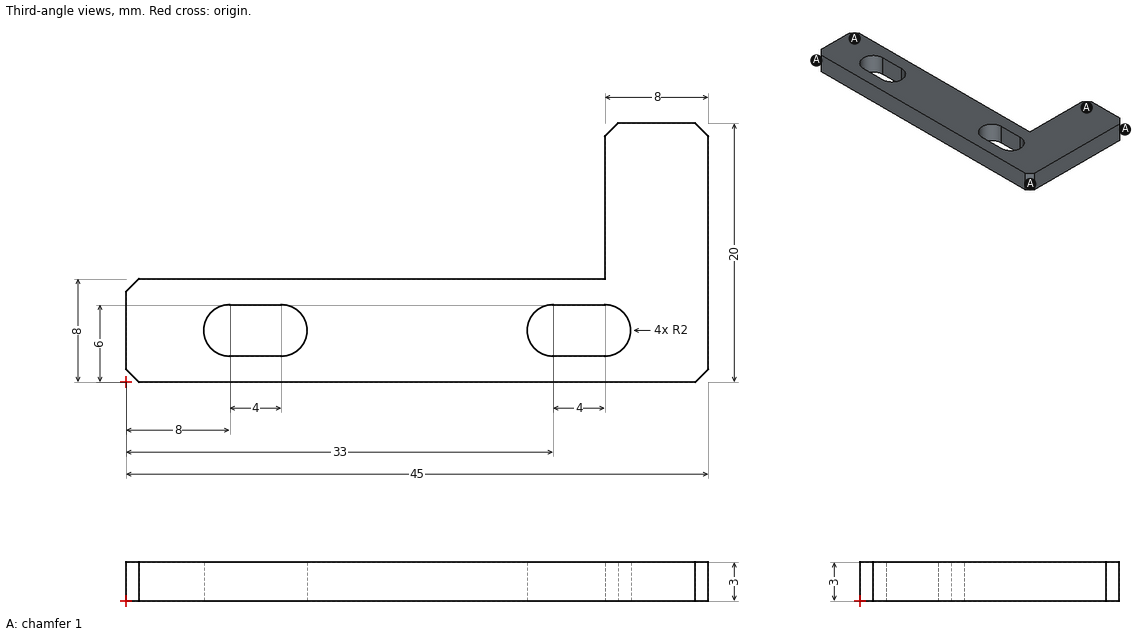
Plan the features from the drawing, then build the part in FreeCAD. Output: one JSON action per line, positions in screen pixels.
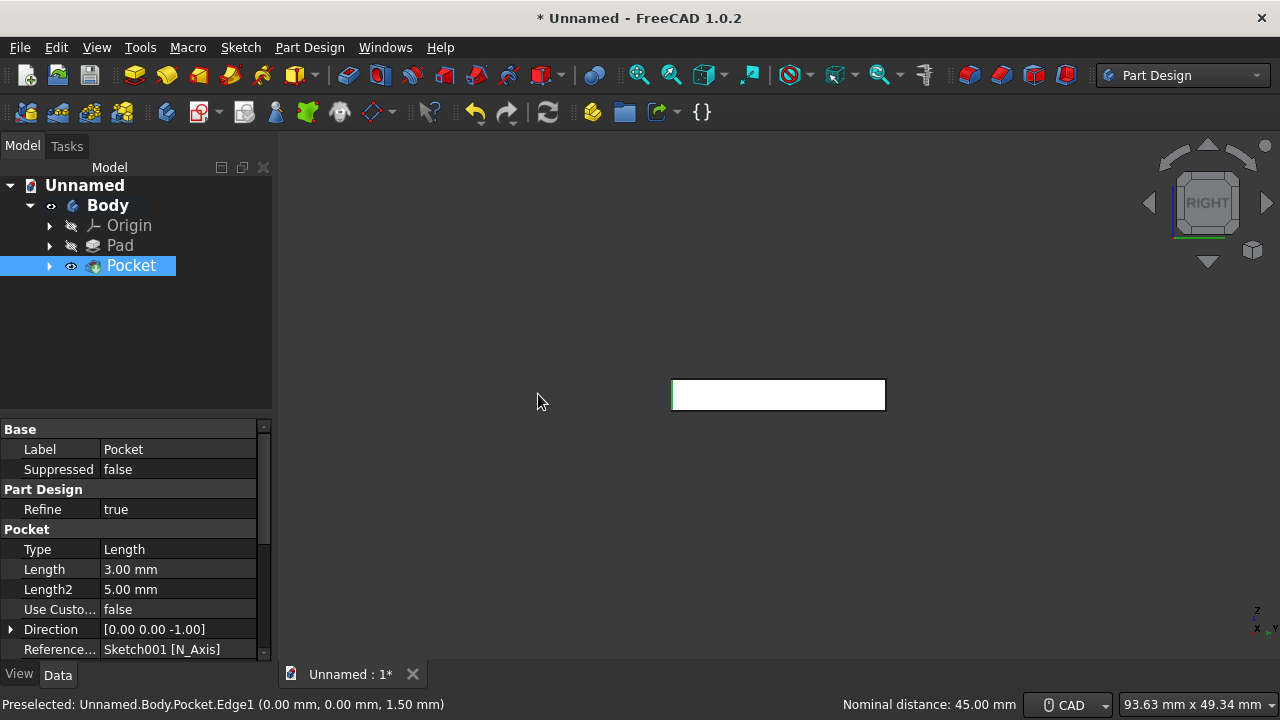
{"action": "left_click", "coordinate": [640, 76]}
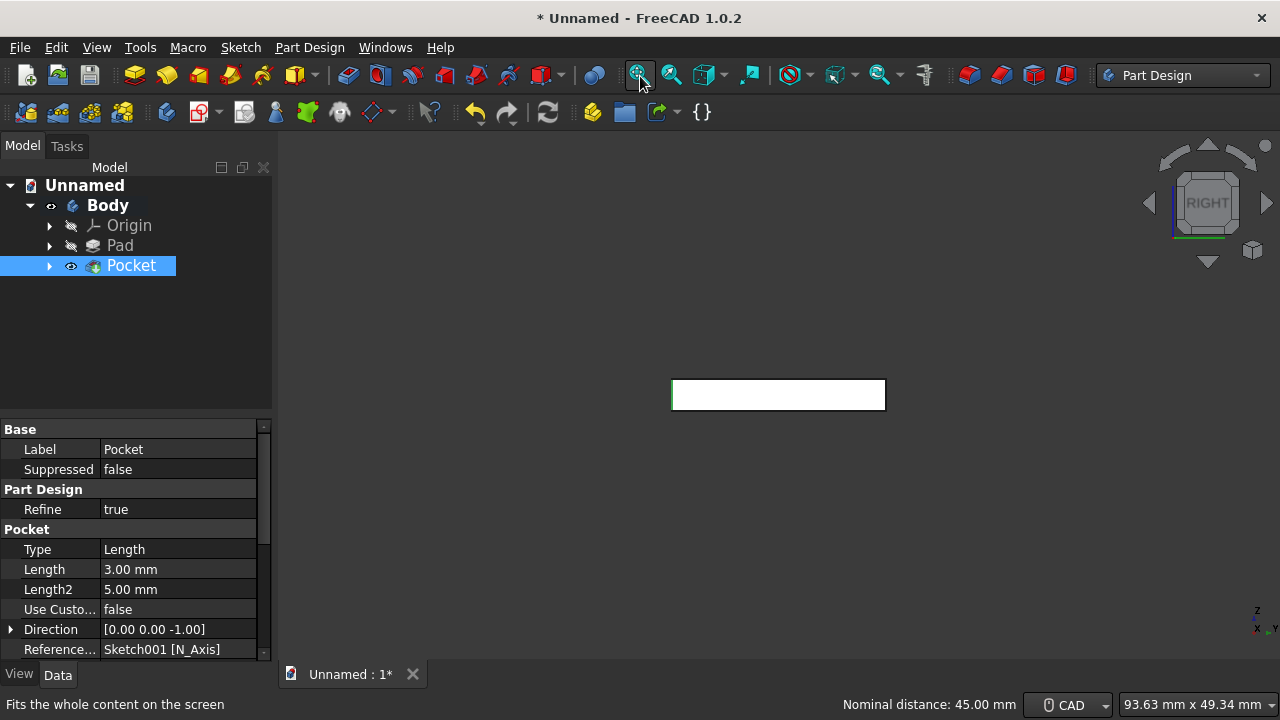
{"action": "left_click", "coordinate": [886, 394], "text": "ctrl"}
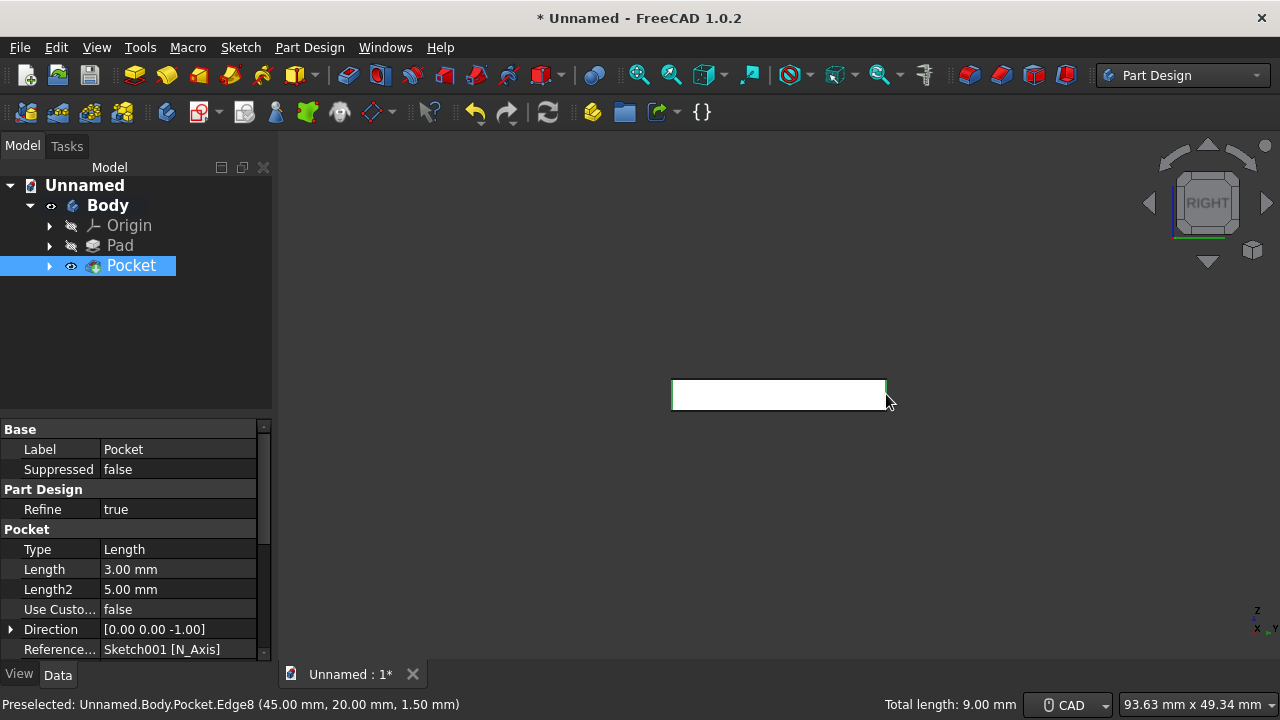
{"action": "key", "text": "5"}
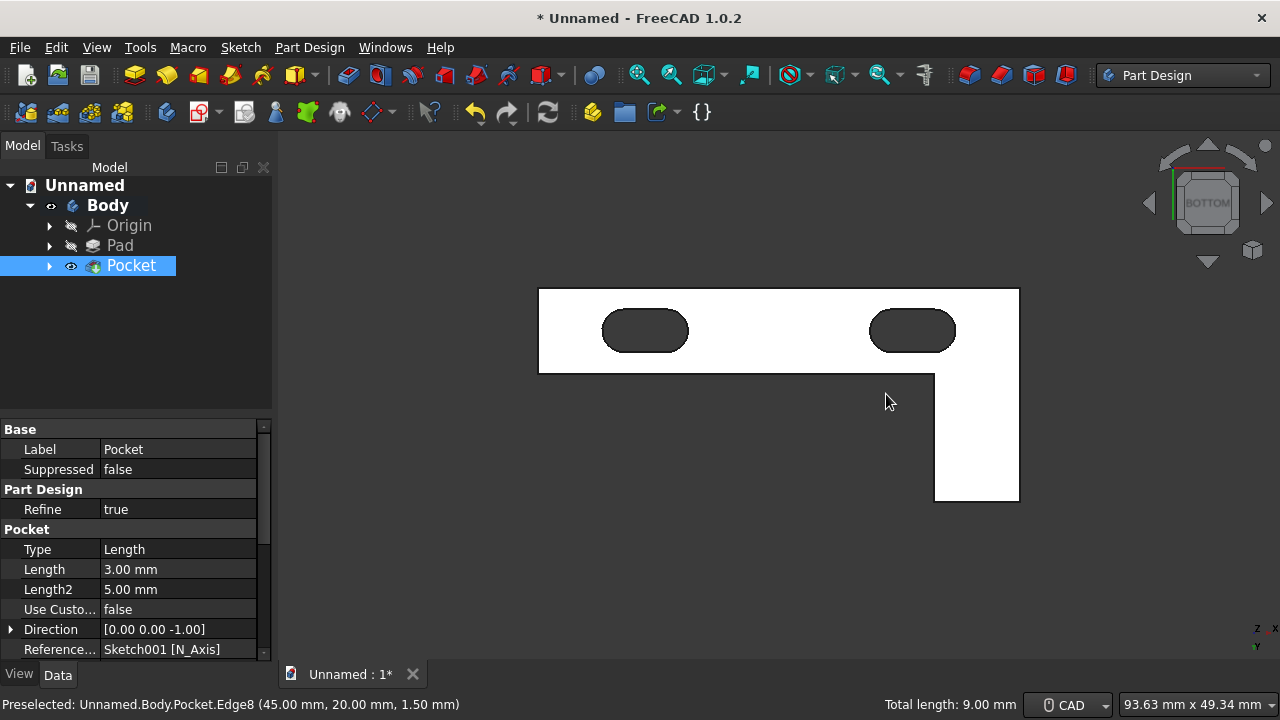
{"action": "key", "text": "4"}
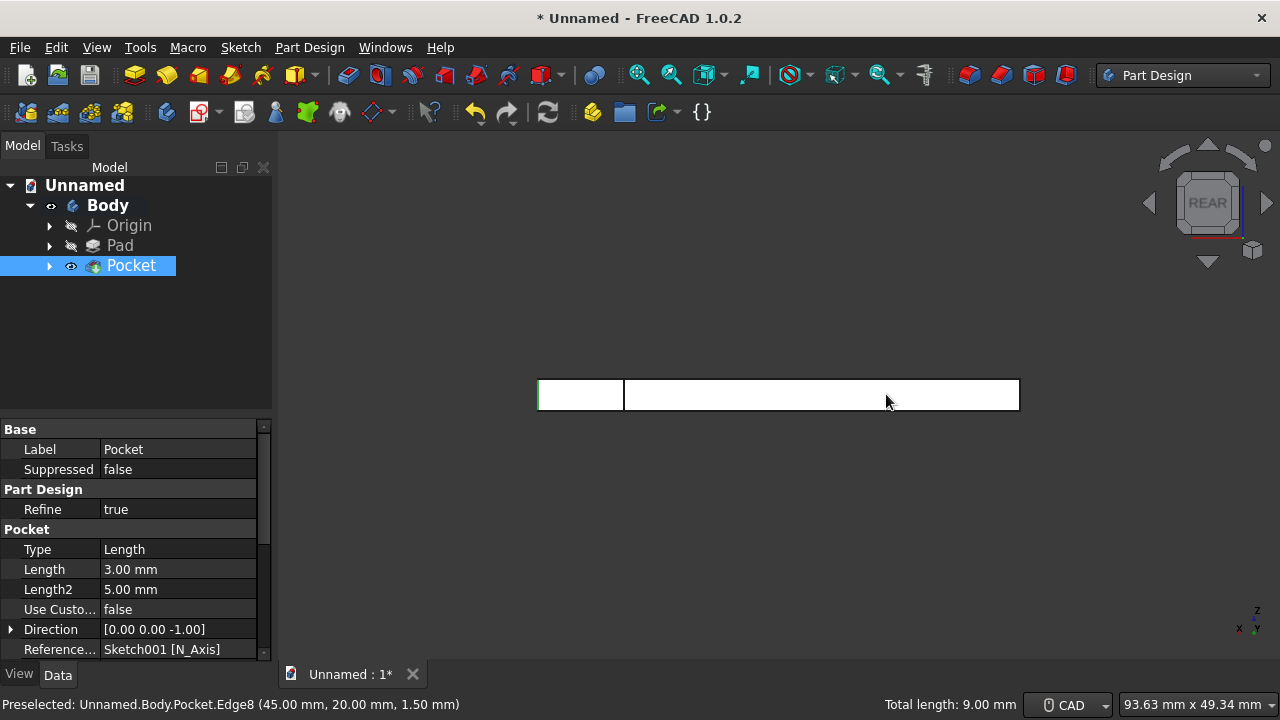
{"action": "left_click", "coordinate": [1020, 394], "text": "ctrl"}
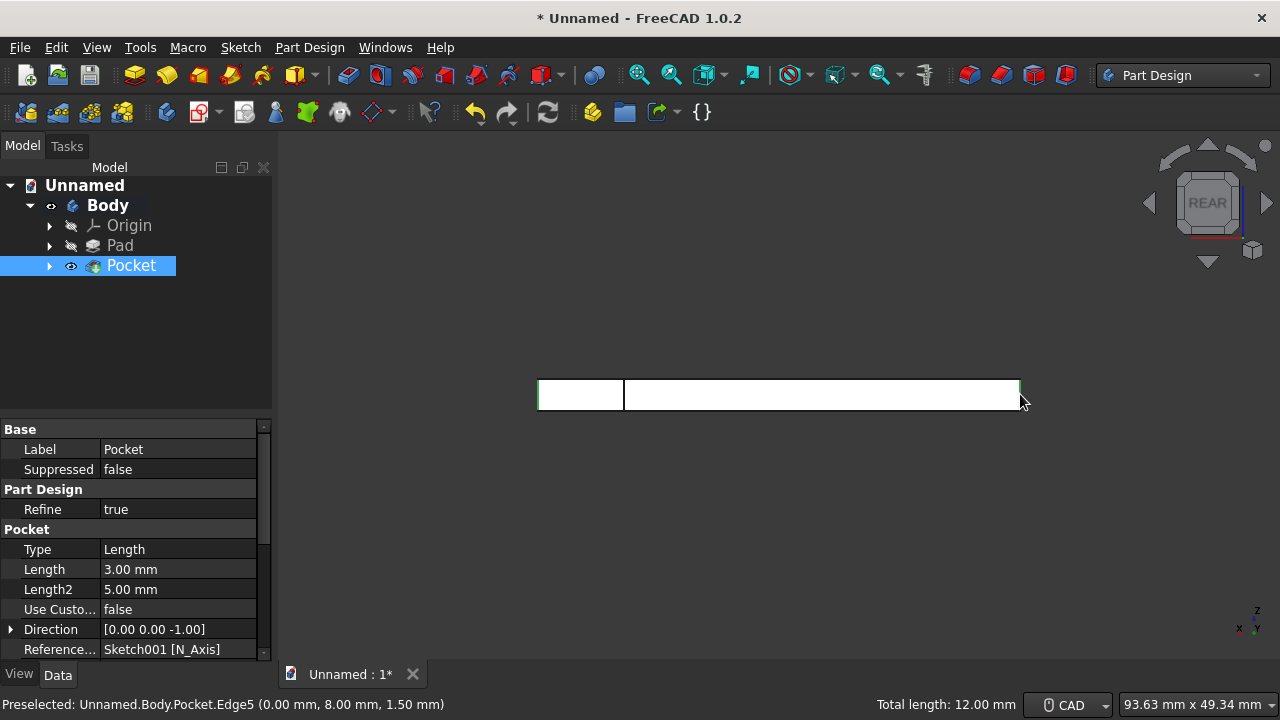
{"action": "left_click", "coordinate": [624, 394], "text": "ctrl"}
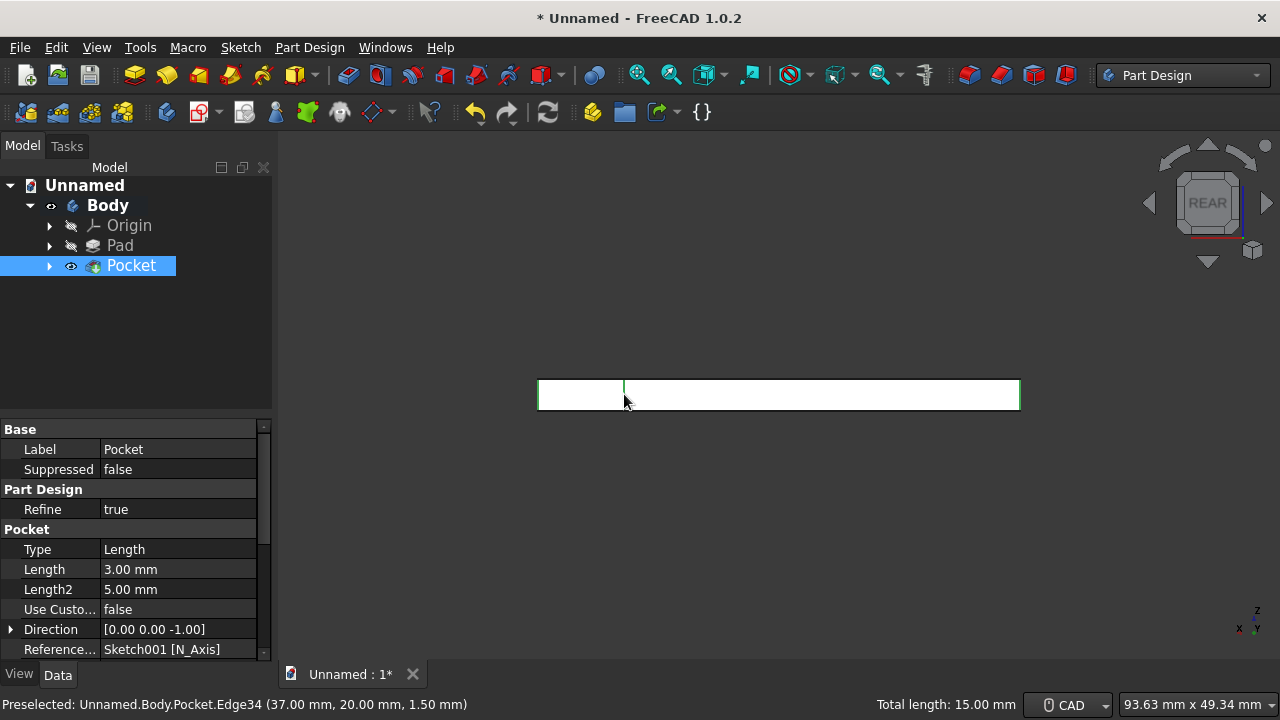
{"action": "left_click", "coordinate": [1002, 76]}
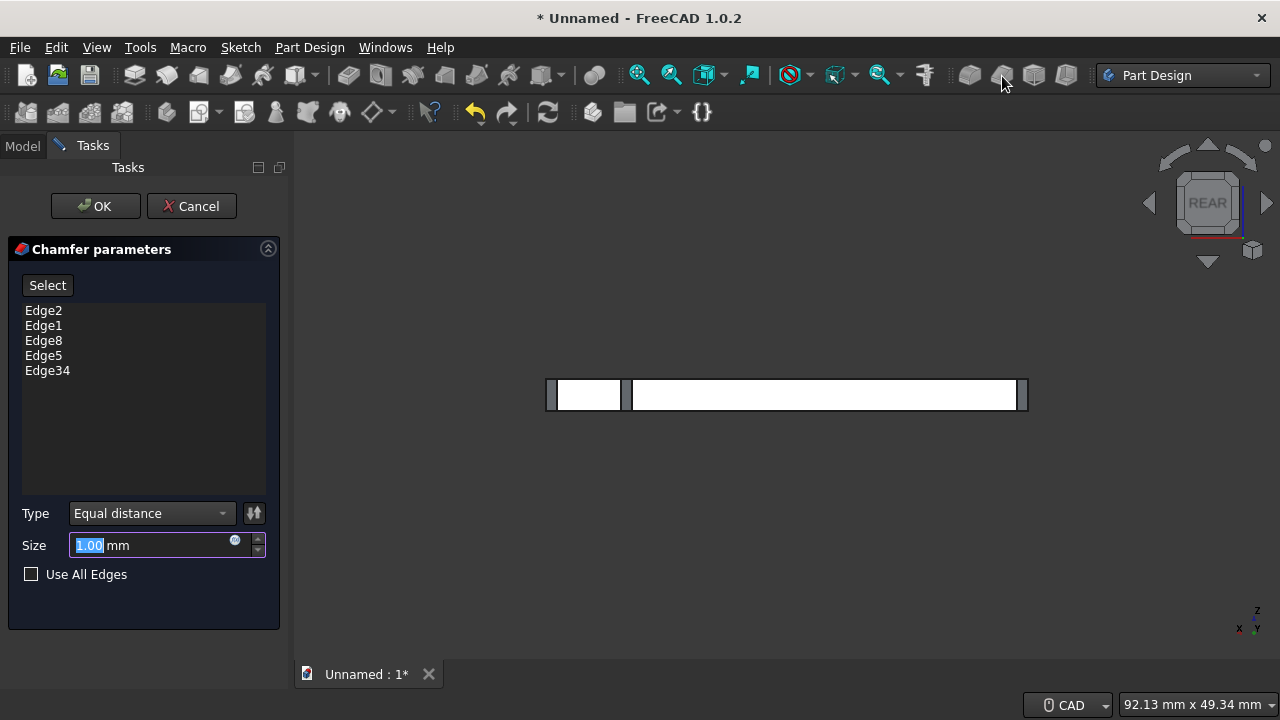
{"action": "type", "text": "1"}
{"action": "key", "text": "Tab"}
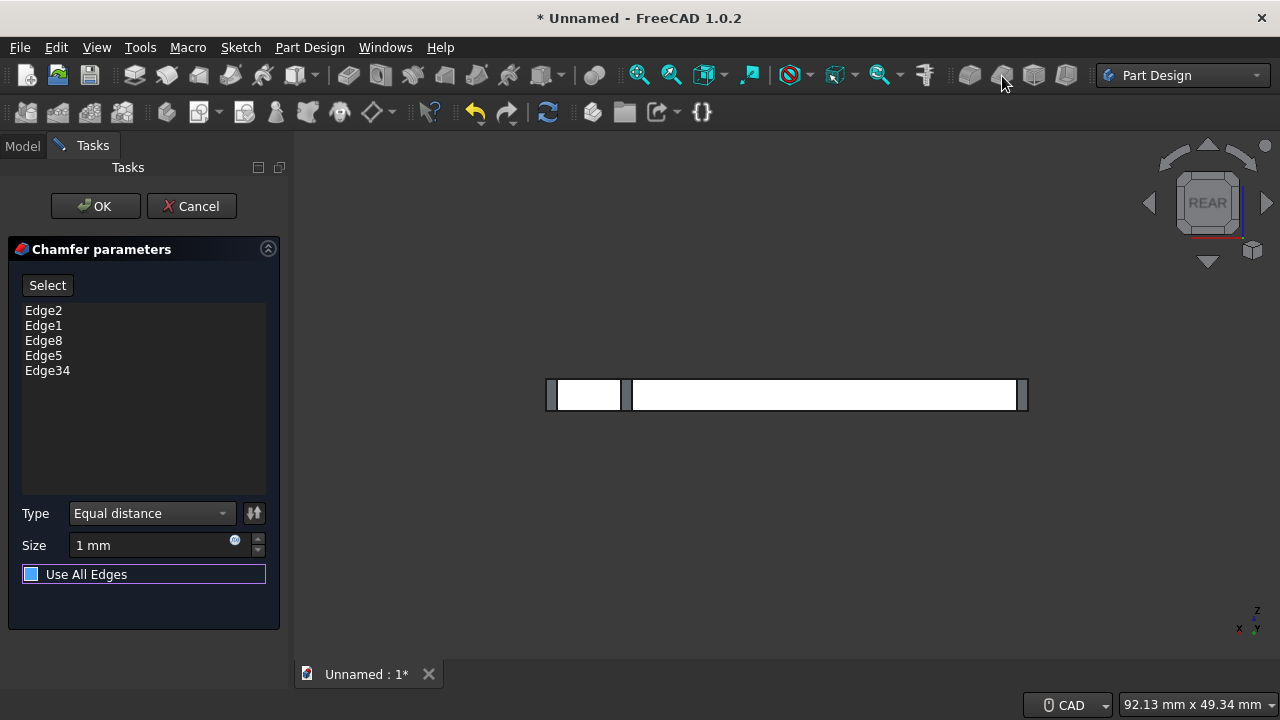
{"action": "left_click", "coordinate": [96, 206]}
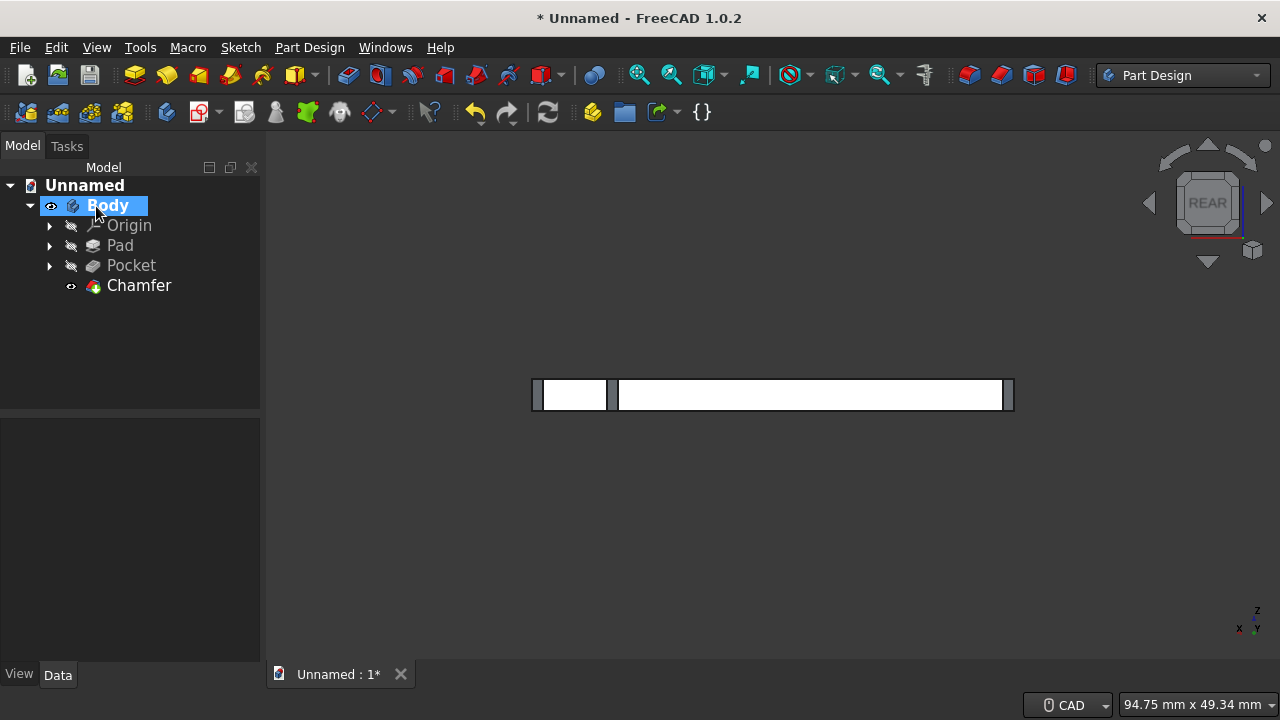
{"action": "key", "text": "0"}